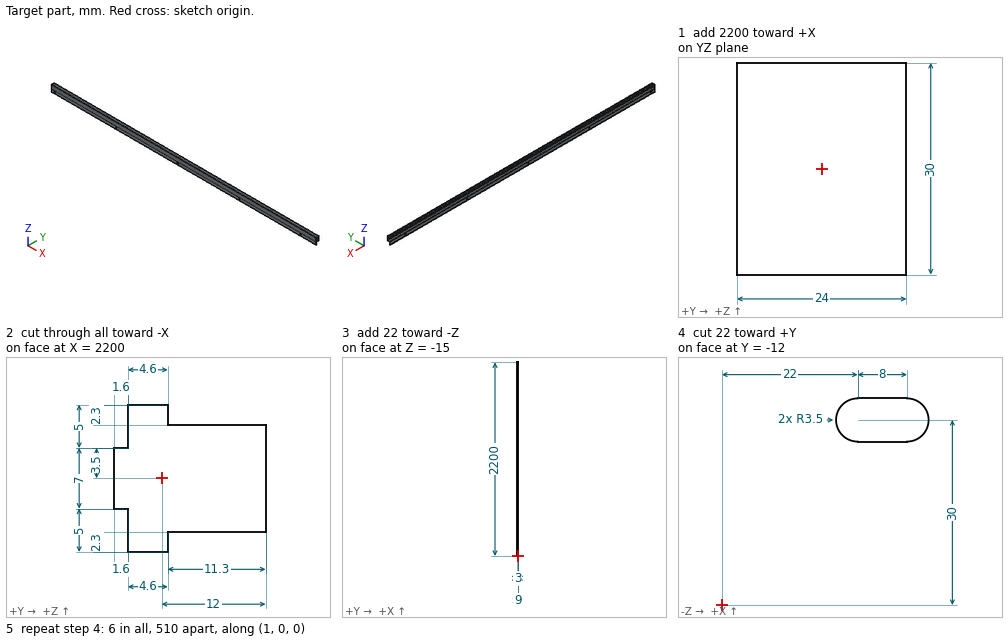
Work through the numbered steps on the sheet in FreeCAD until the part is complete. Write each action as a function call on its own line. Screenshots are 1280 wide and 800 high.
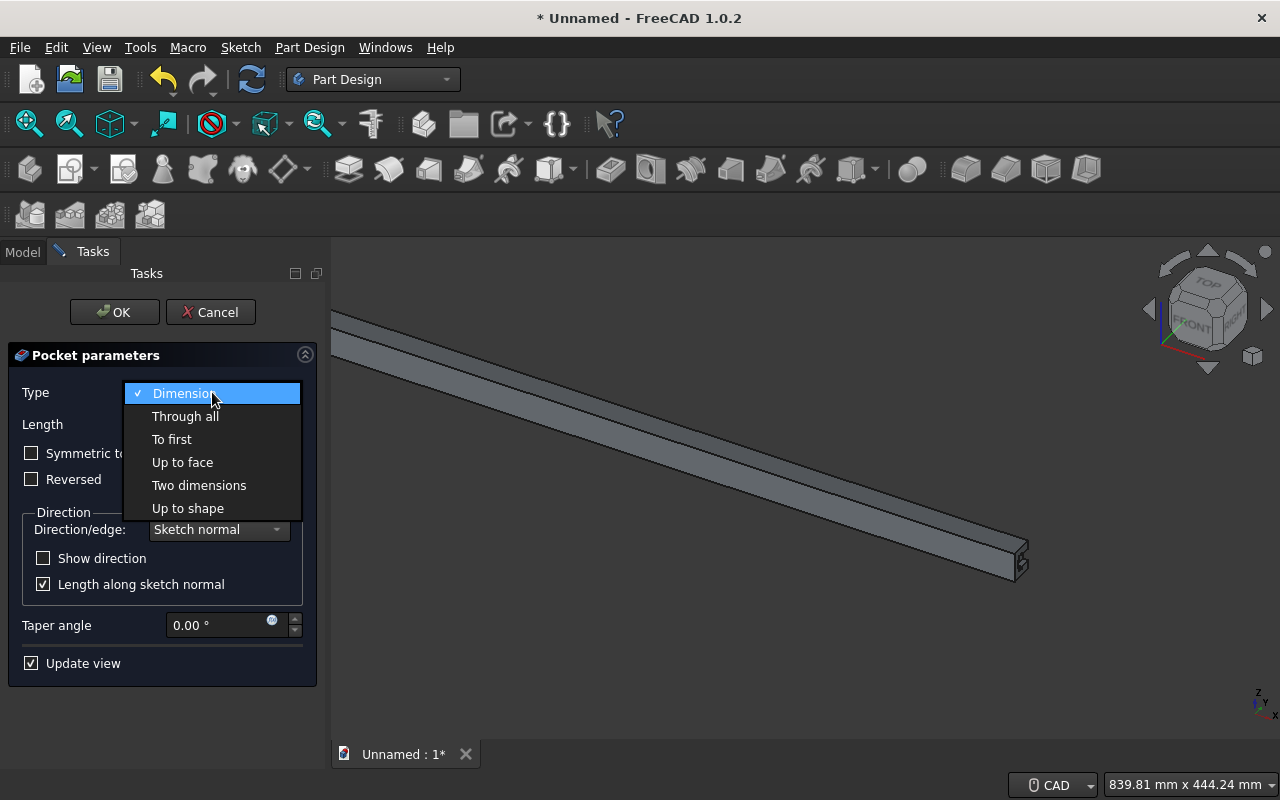
click(212, 416)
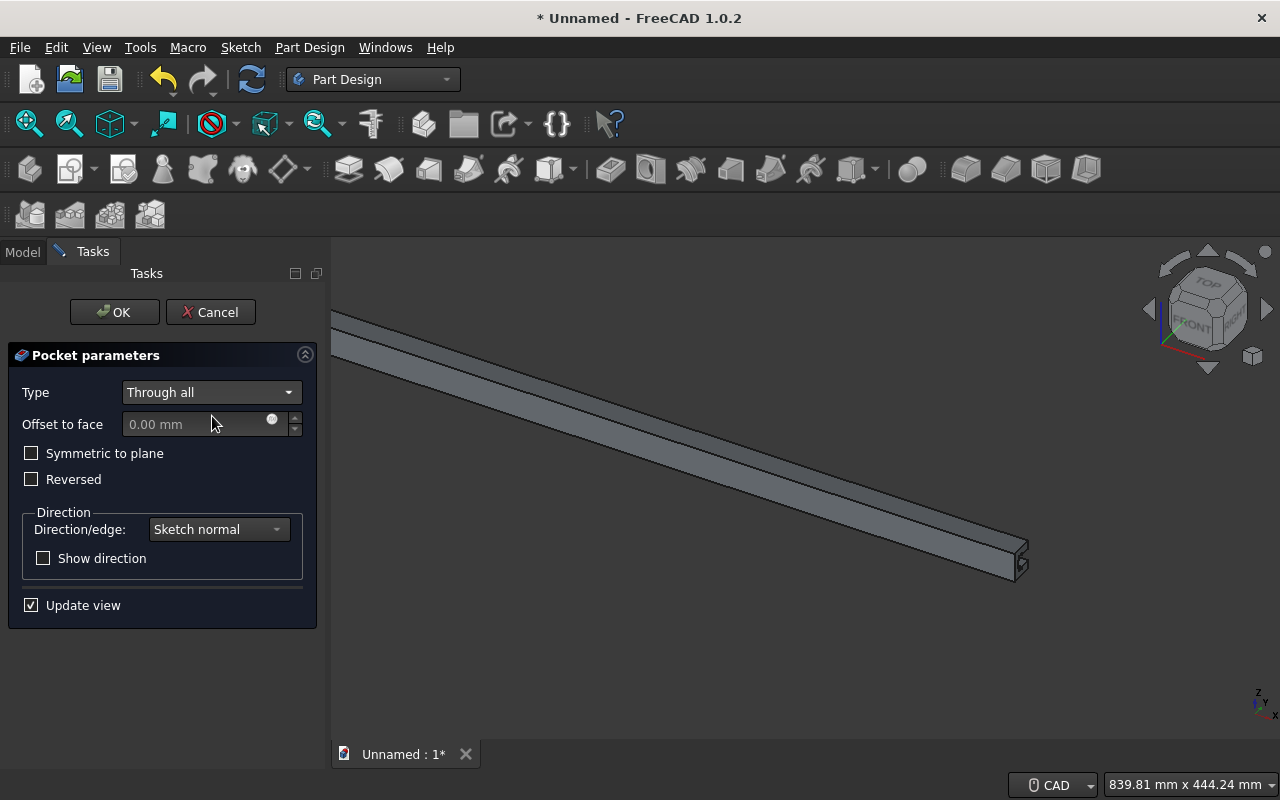
click(115, 312)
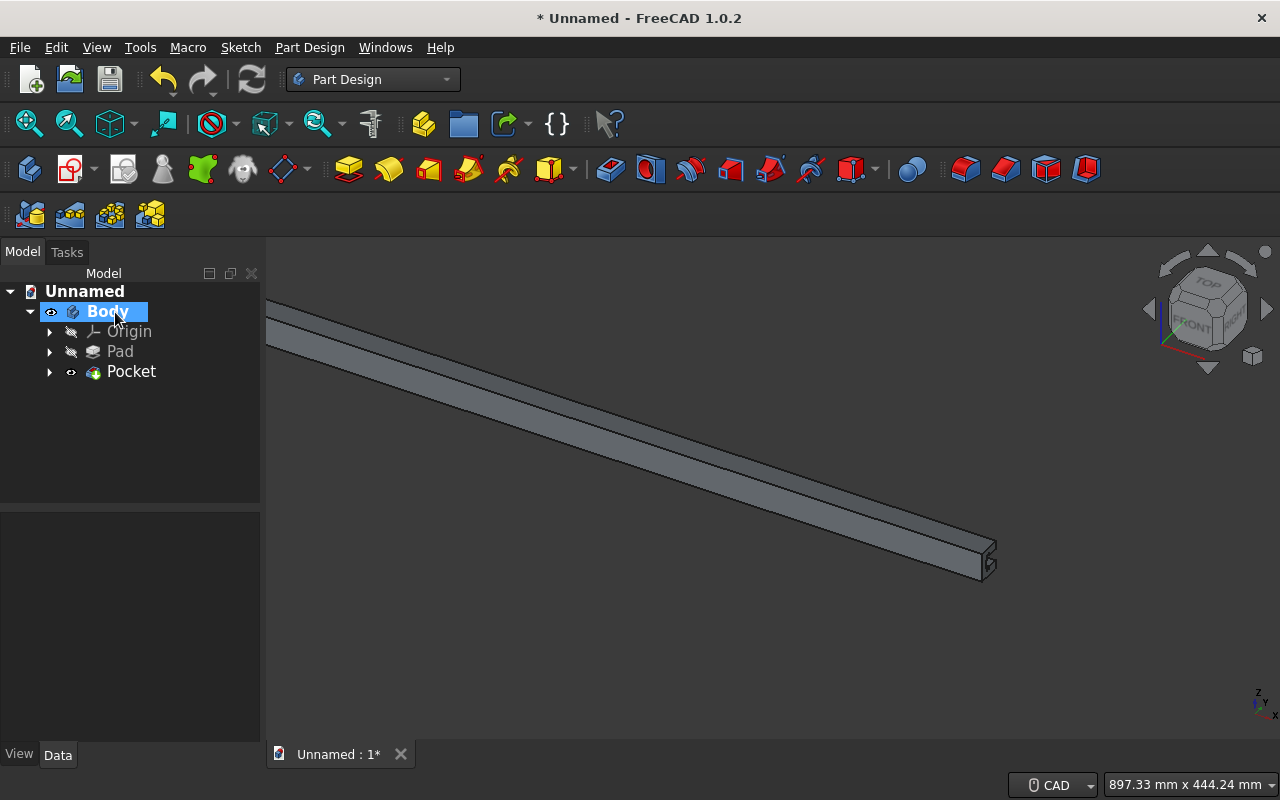
key(v)
key(f)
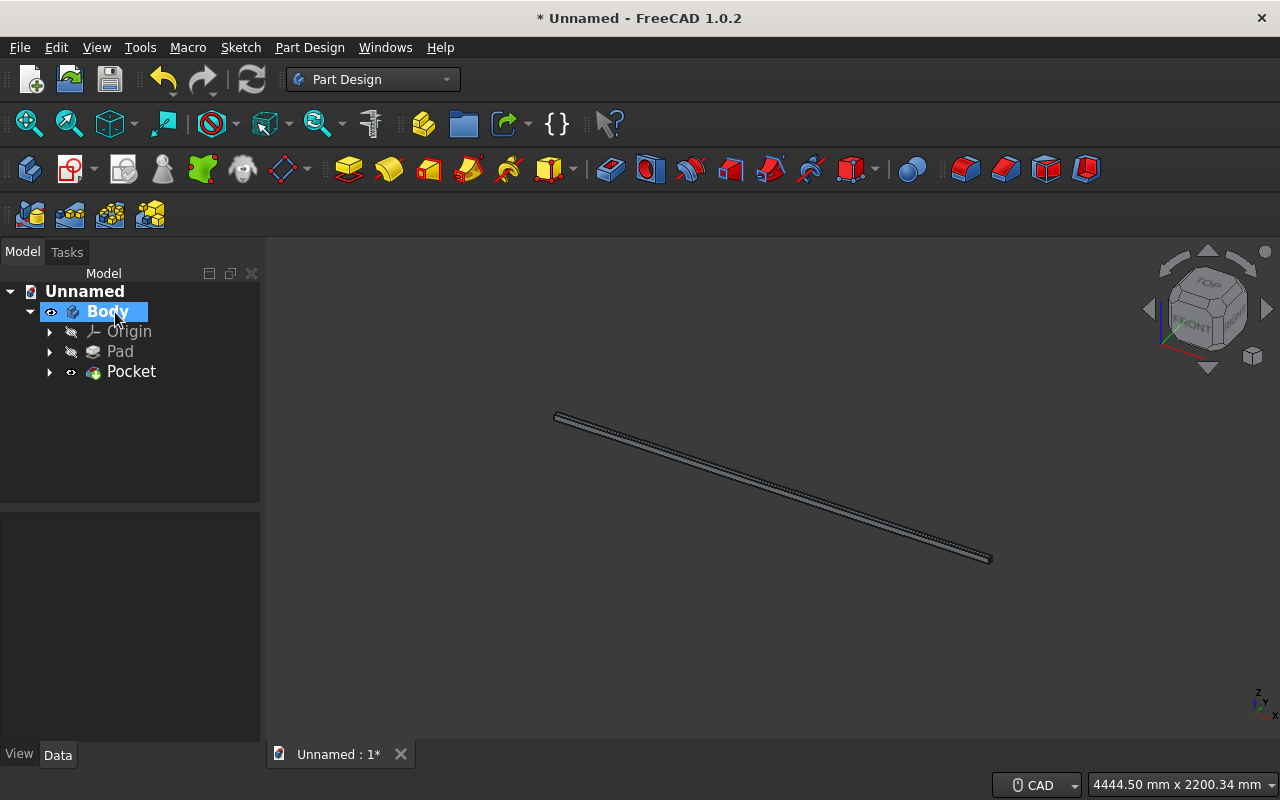
key(5)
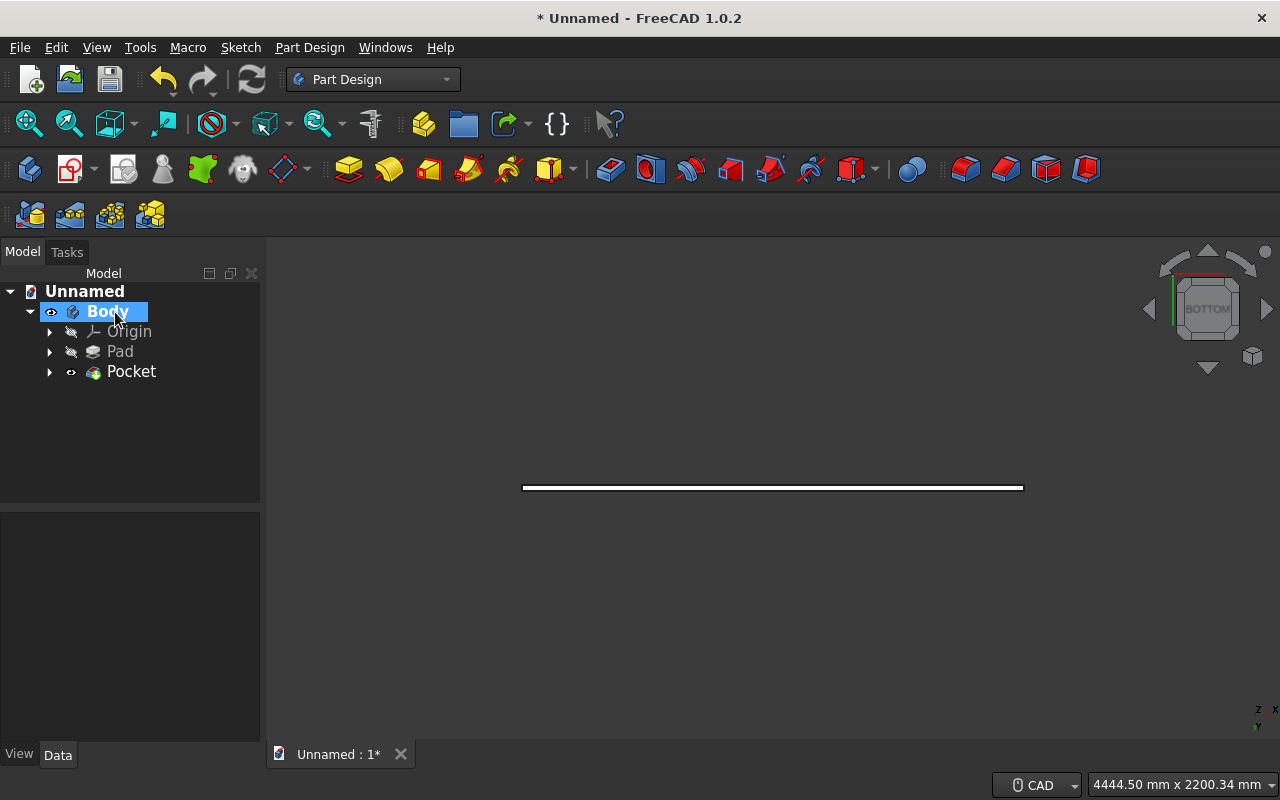
scroll(773, 487, up, 8)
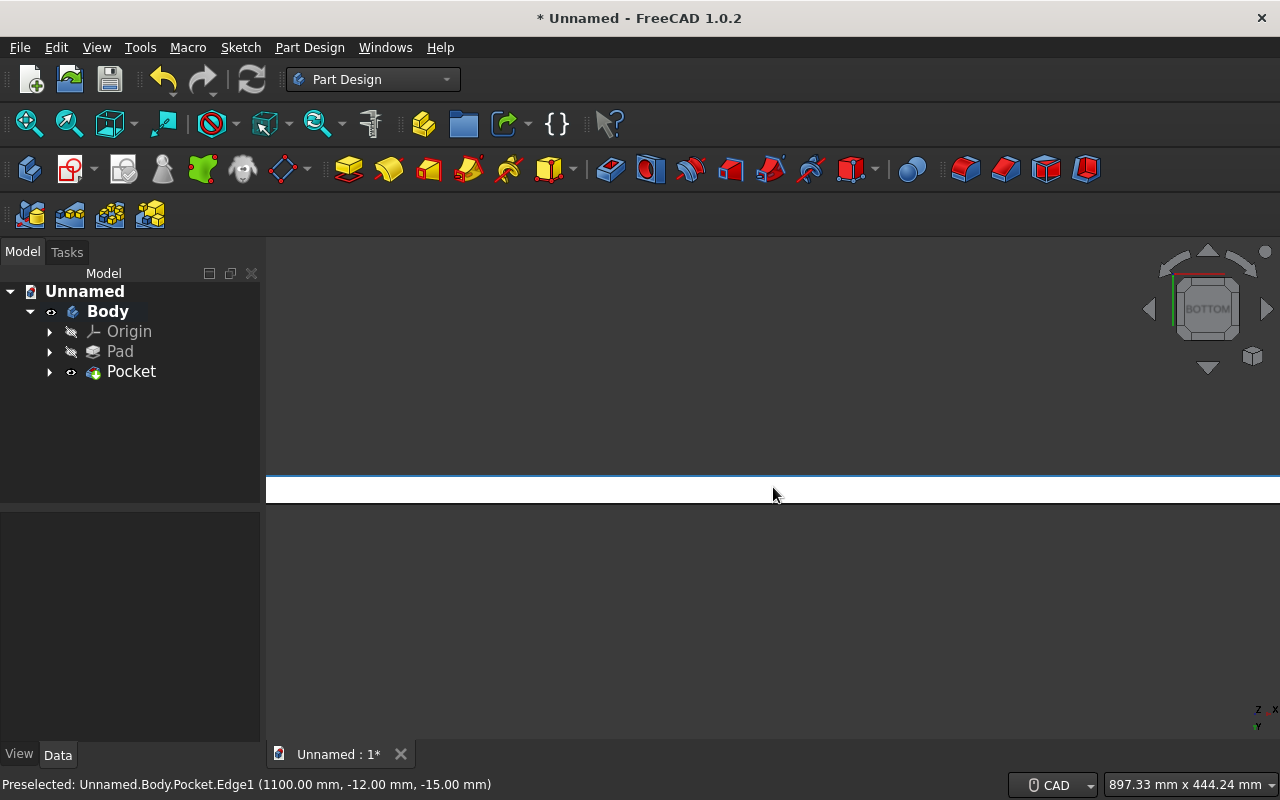
click(771, 489)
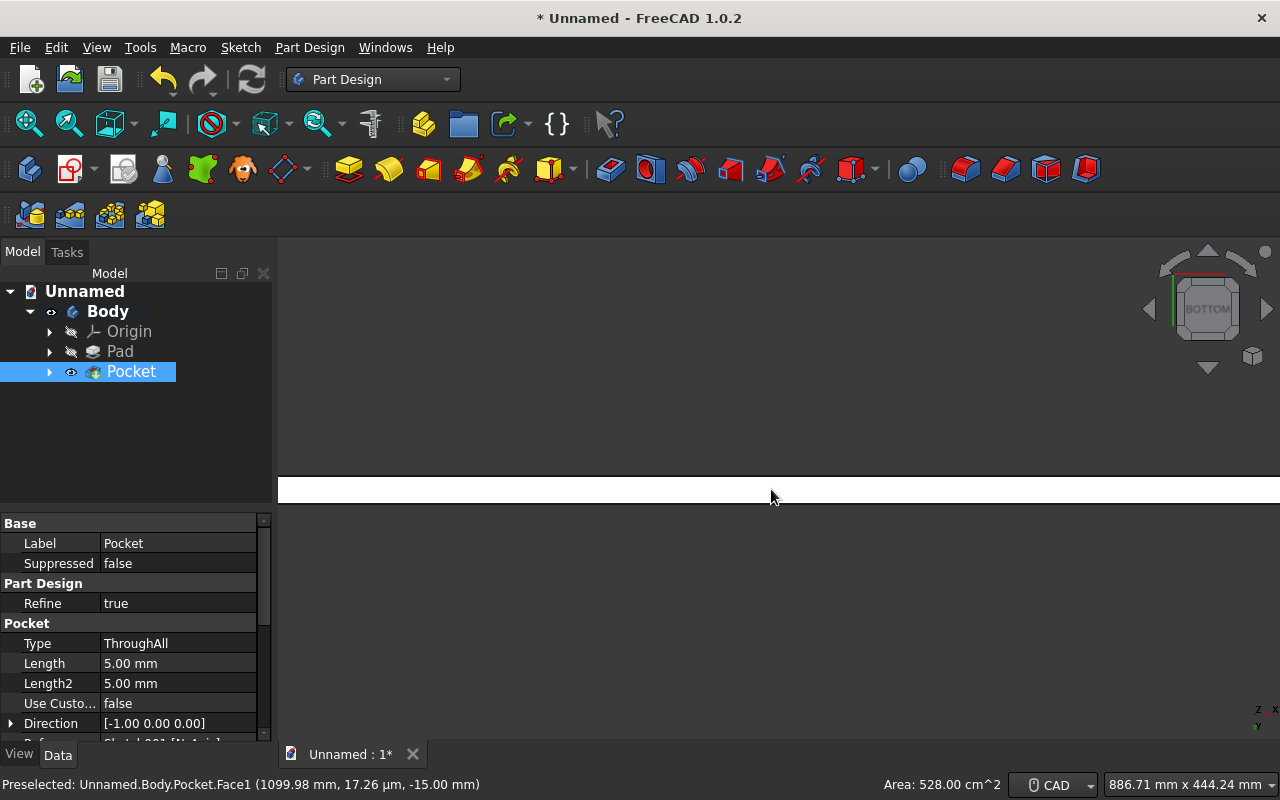
click(70, 170)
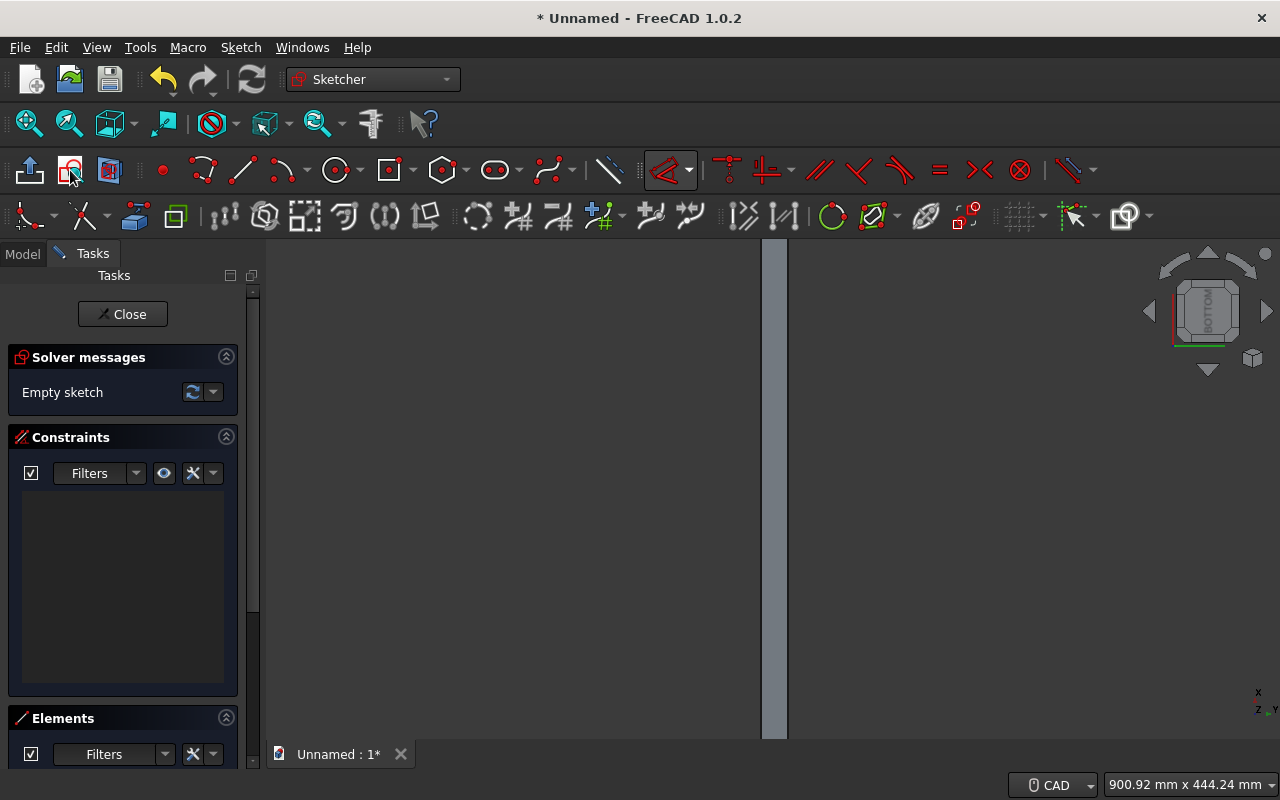
scroll(695, 489, down, 10)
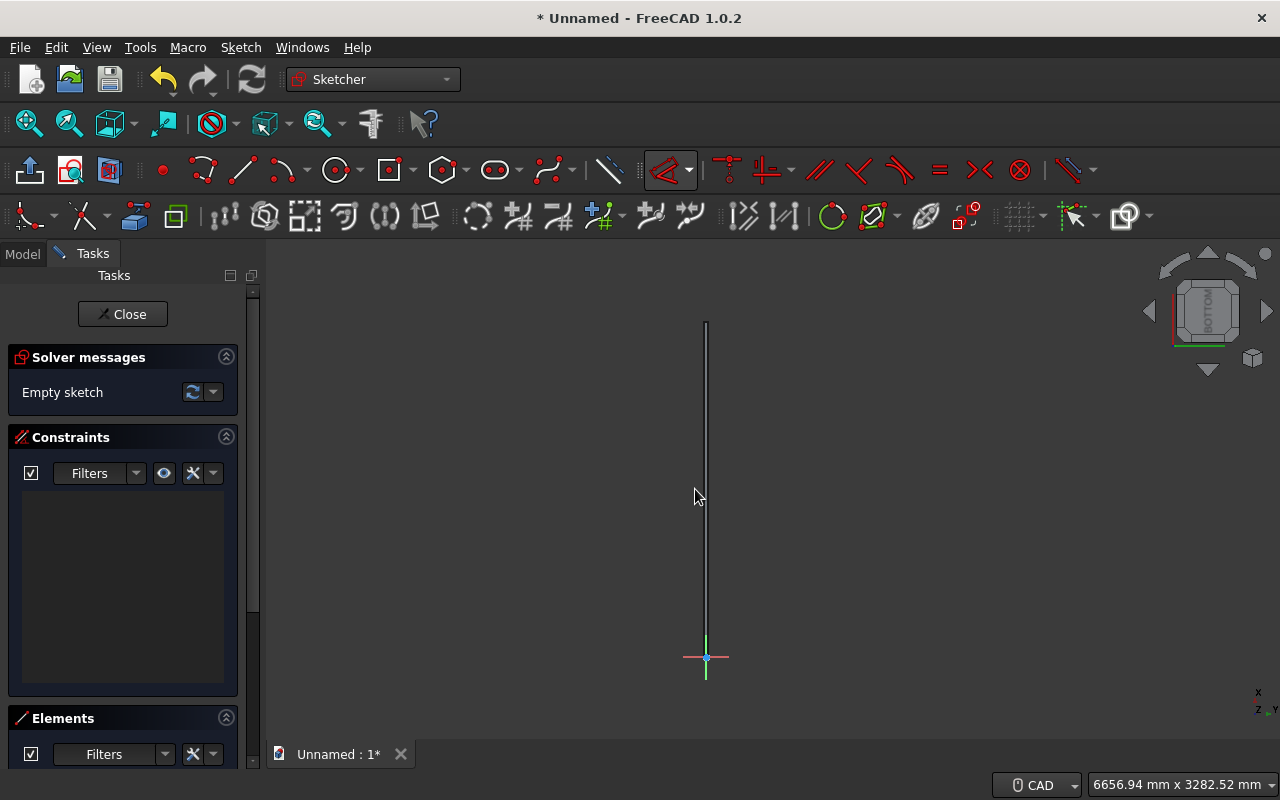
click(416, 170)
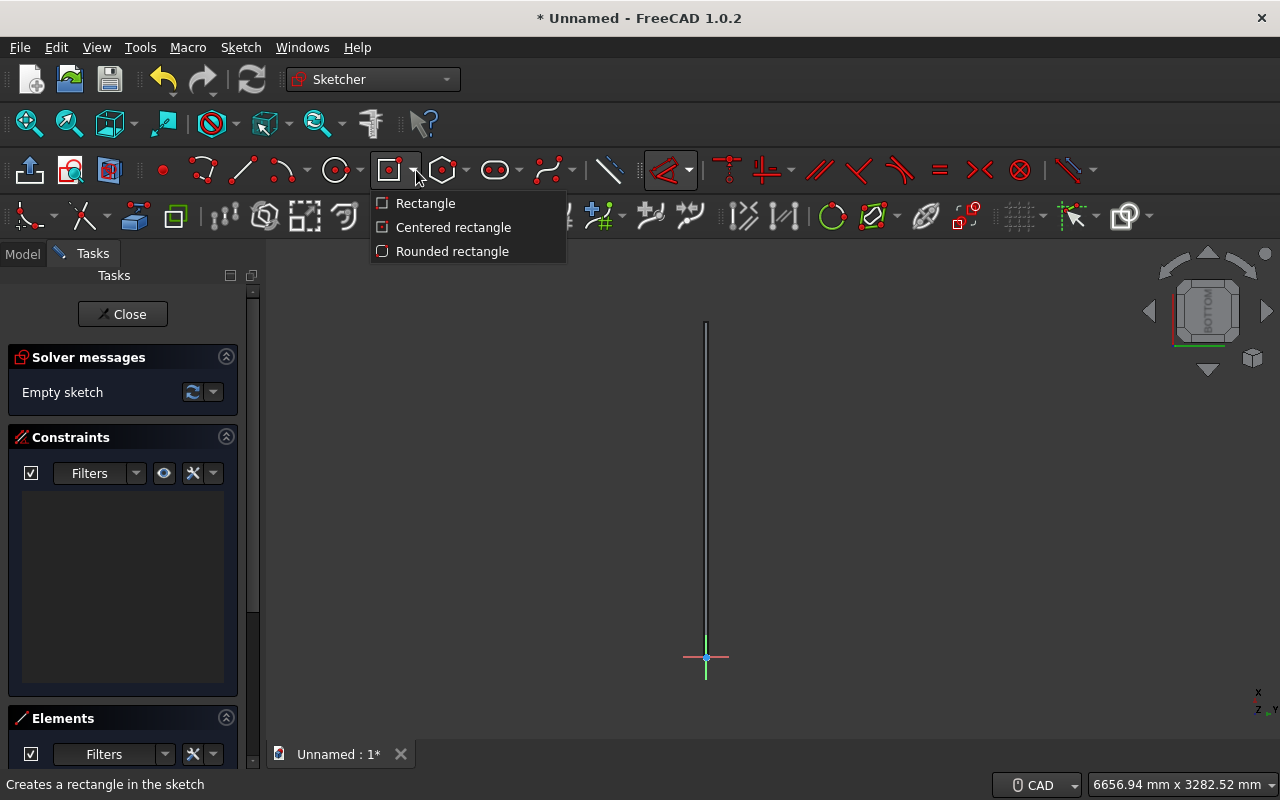
click(468, 203)